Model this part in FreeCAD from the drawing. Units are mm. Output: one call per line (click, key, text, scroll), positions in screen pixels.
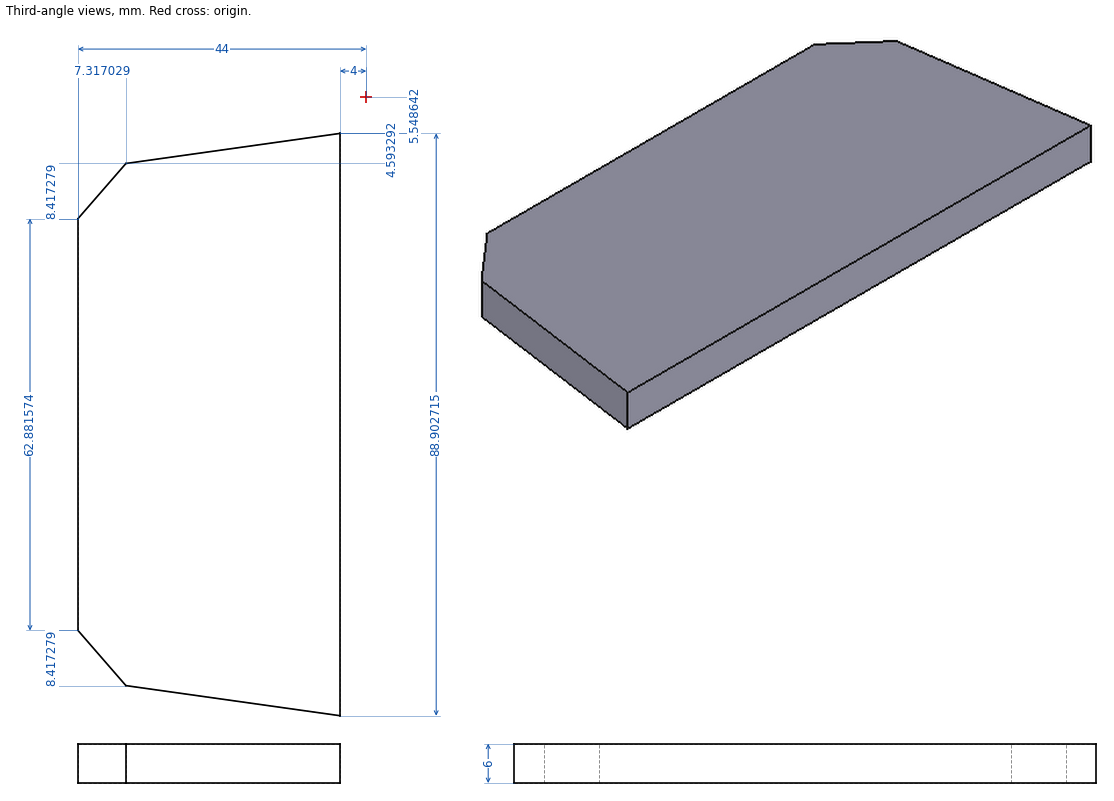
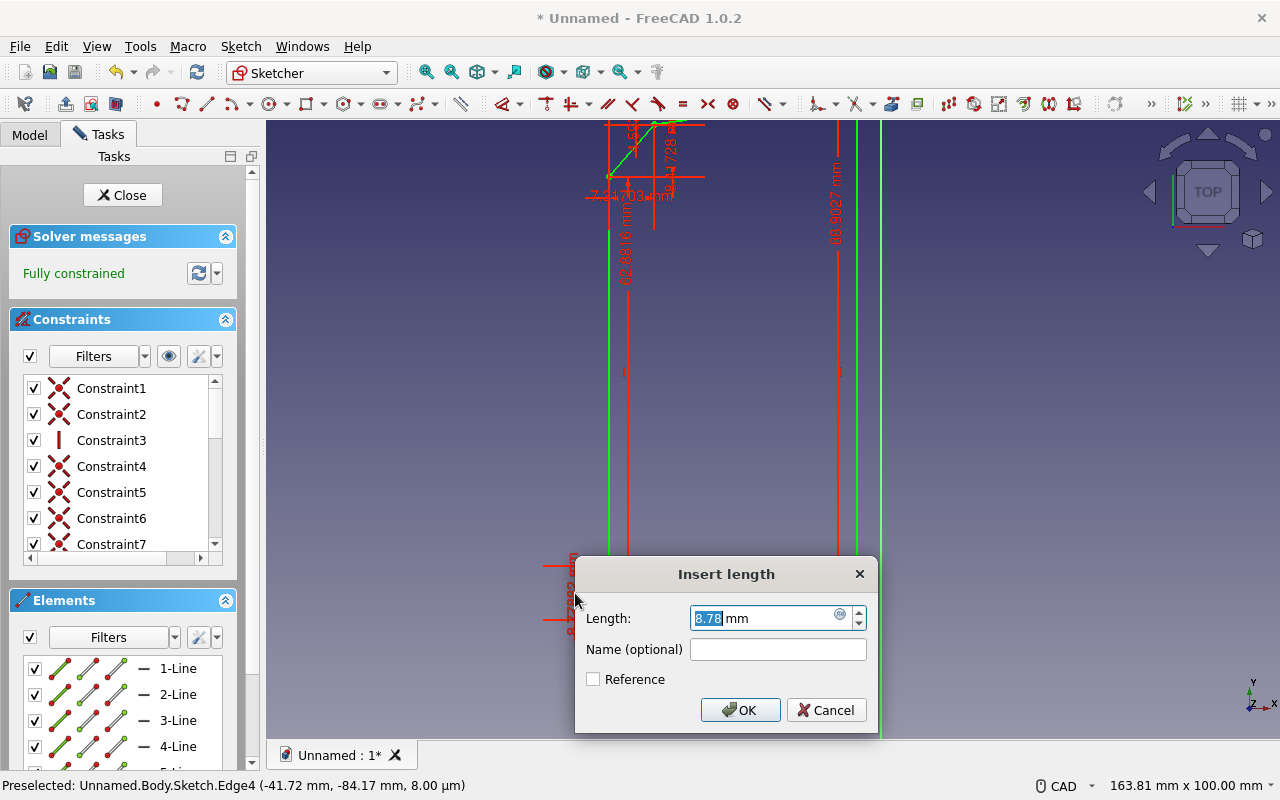
text(8.417279)
key(Return)
key(Escape)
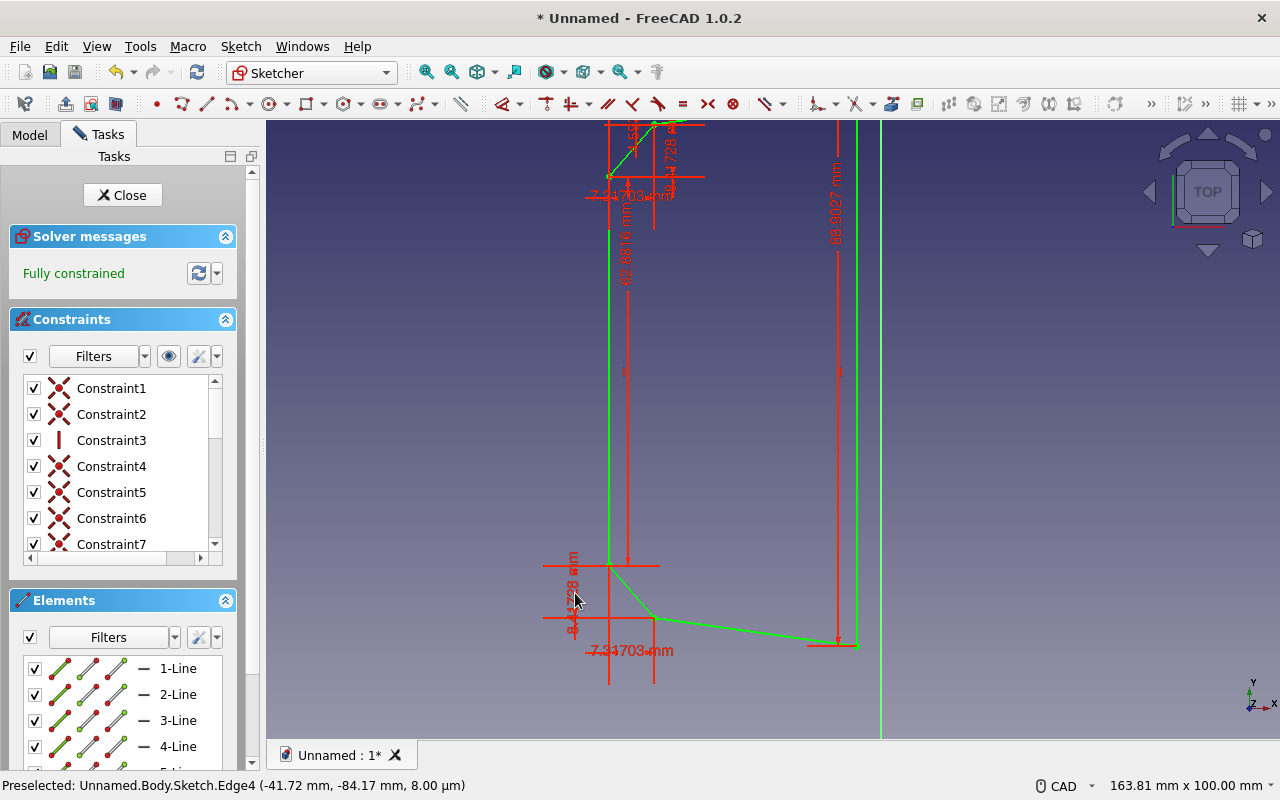
click(123, 195)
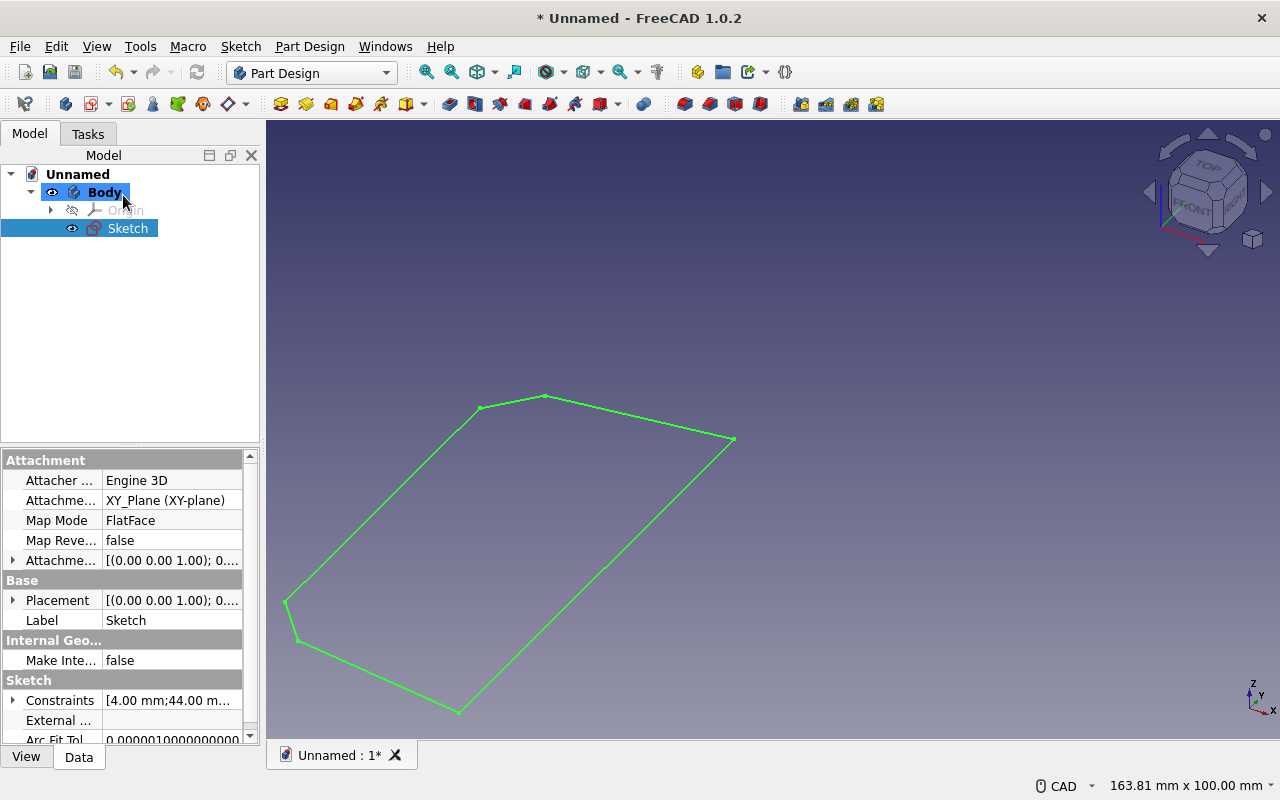
click(281, 104)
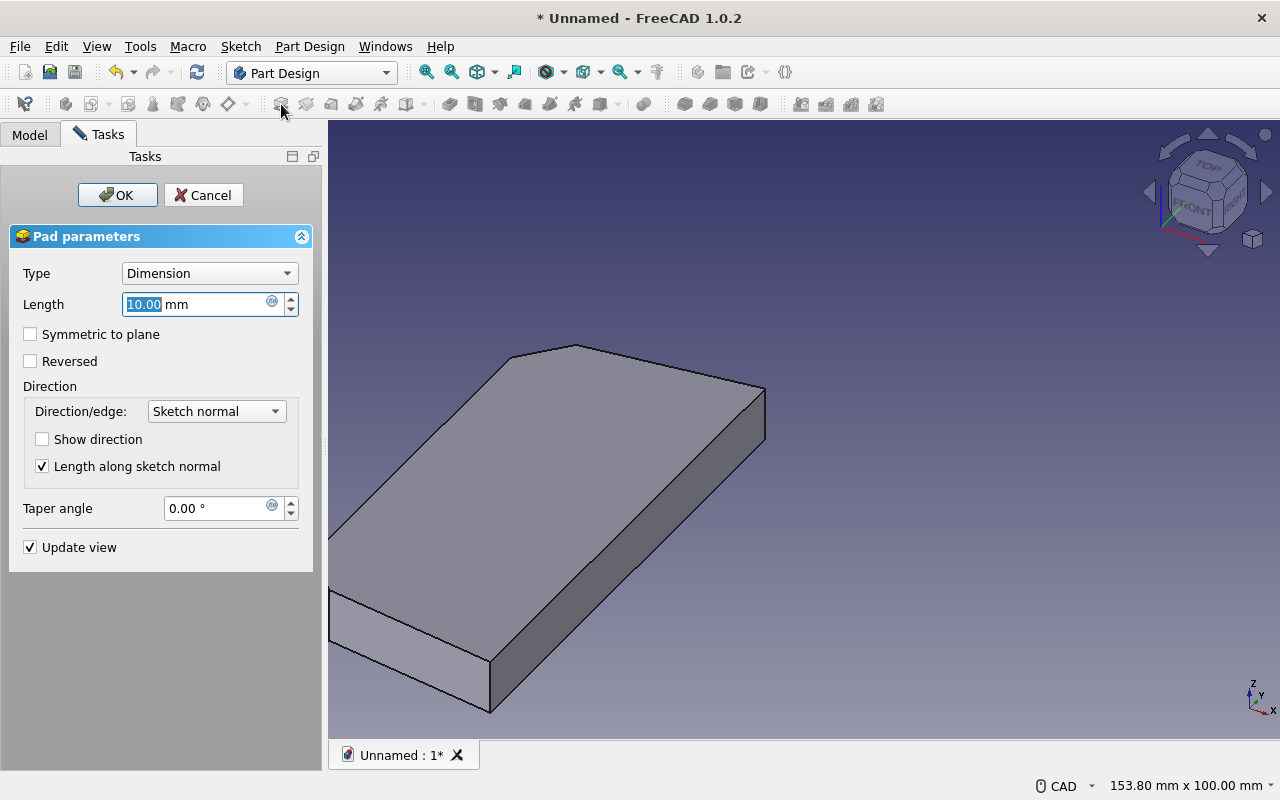
text(6)
key(Tab)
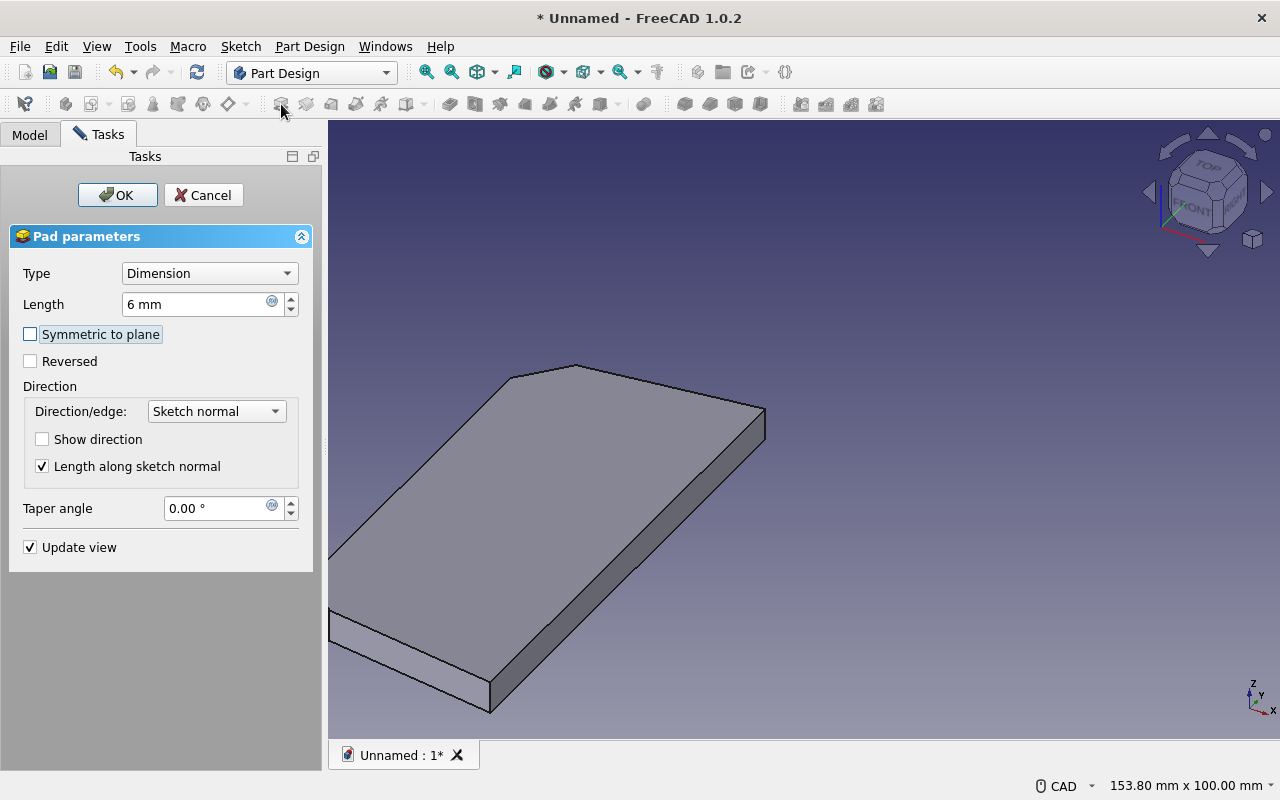
click(118, 195)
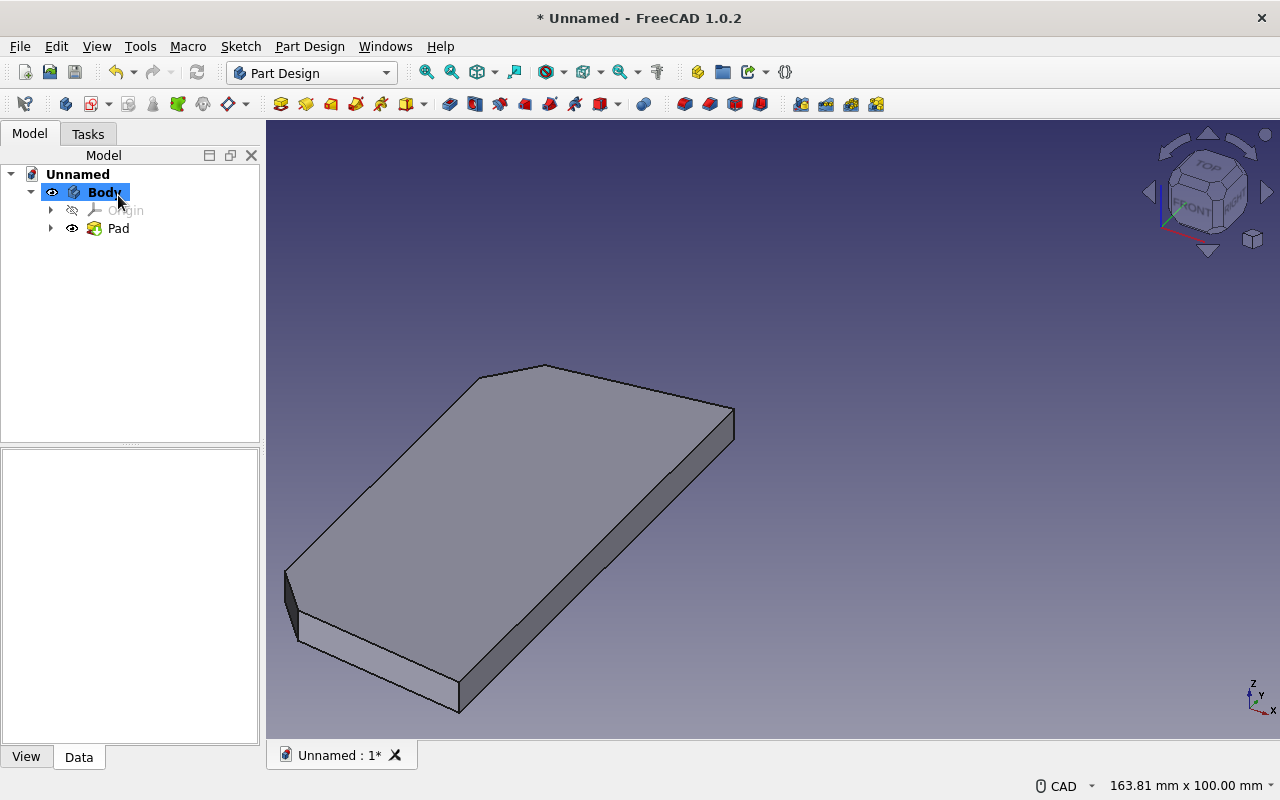
key(0)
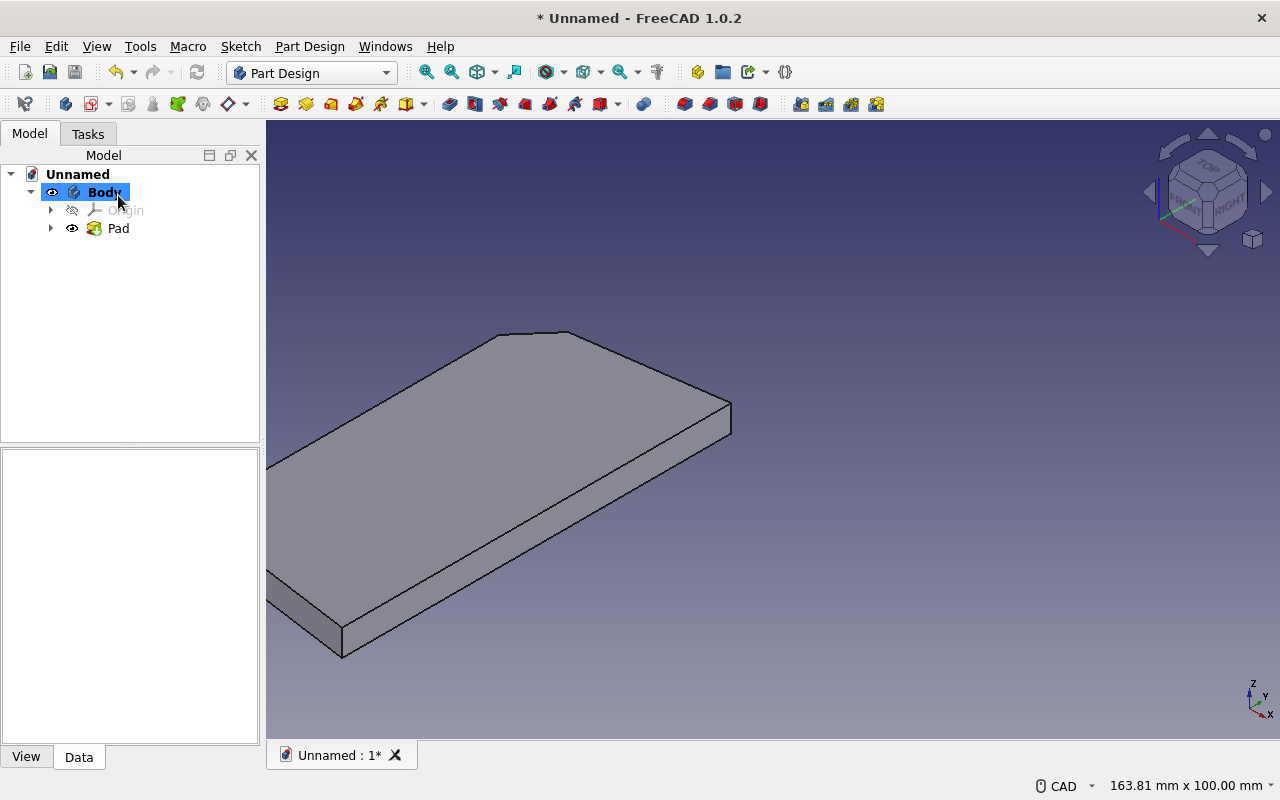
click(427, 72)